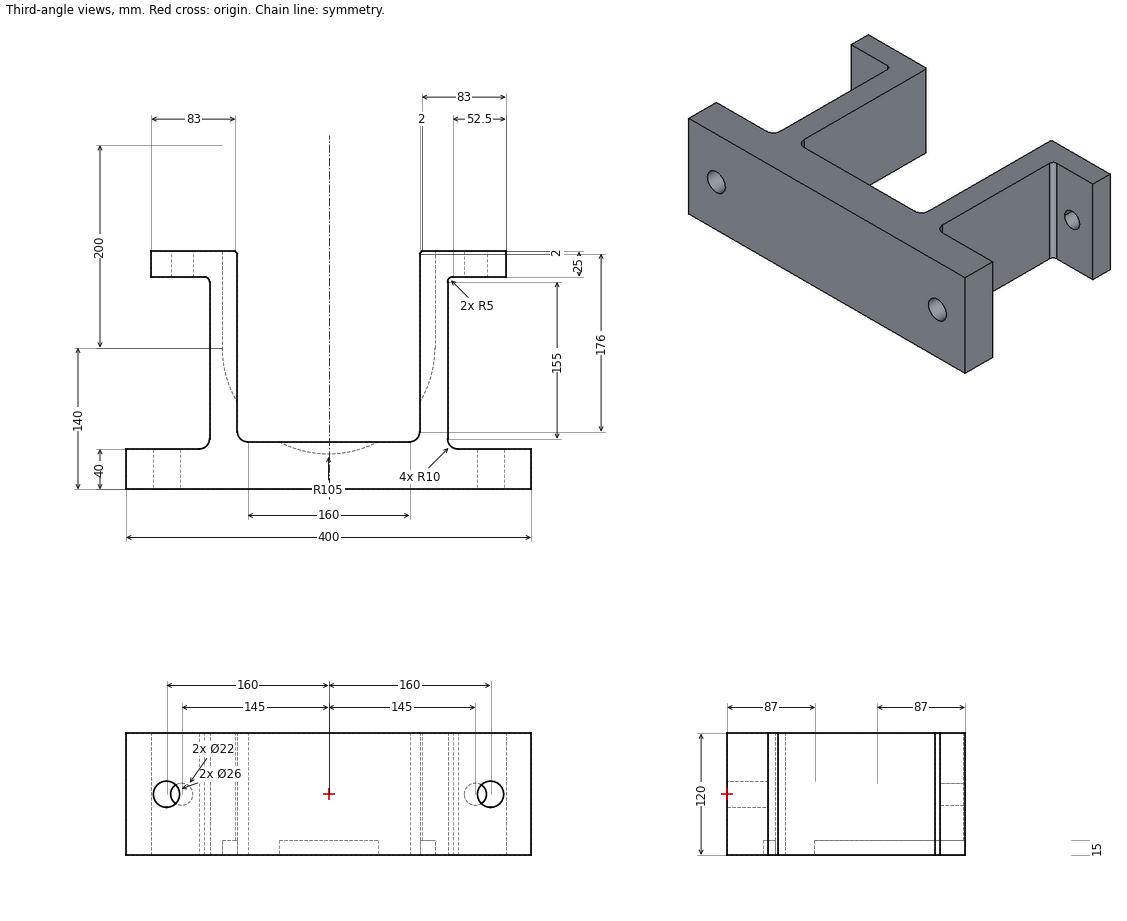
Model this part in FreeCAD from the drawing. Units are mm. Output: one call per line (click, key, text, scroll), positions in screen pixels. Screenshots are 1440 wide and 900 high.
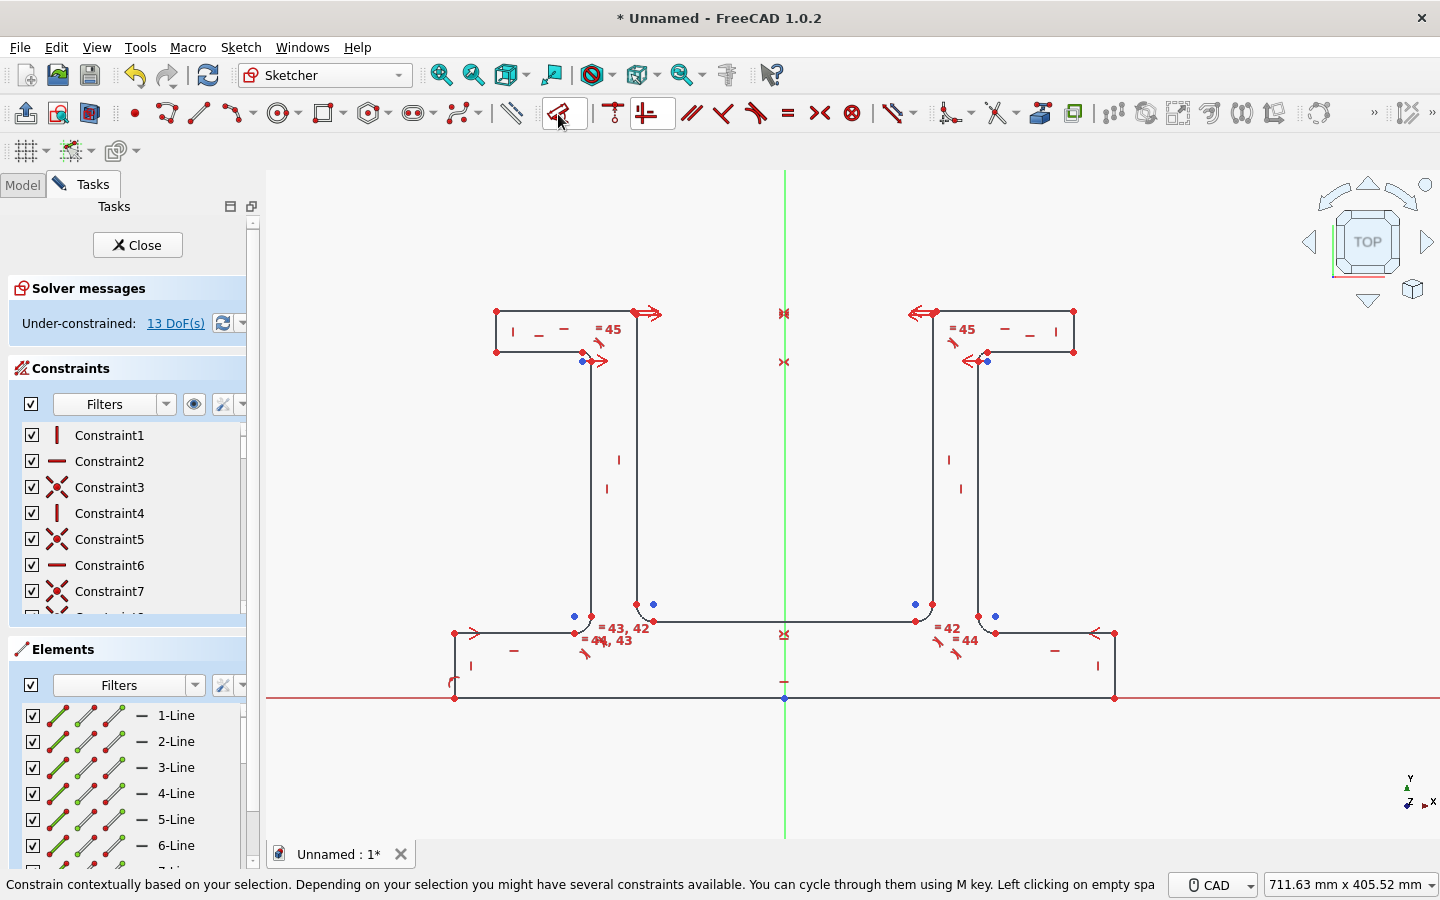
scroll(981, 355, up, 8)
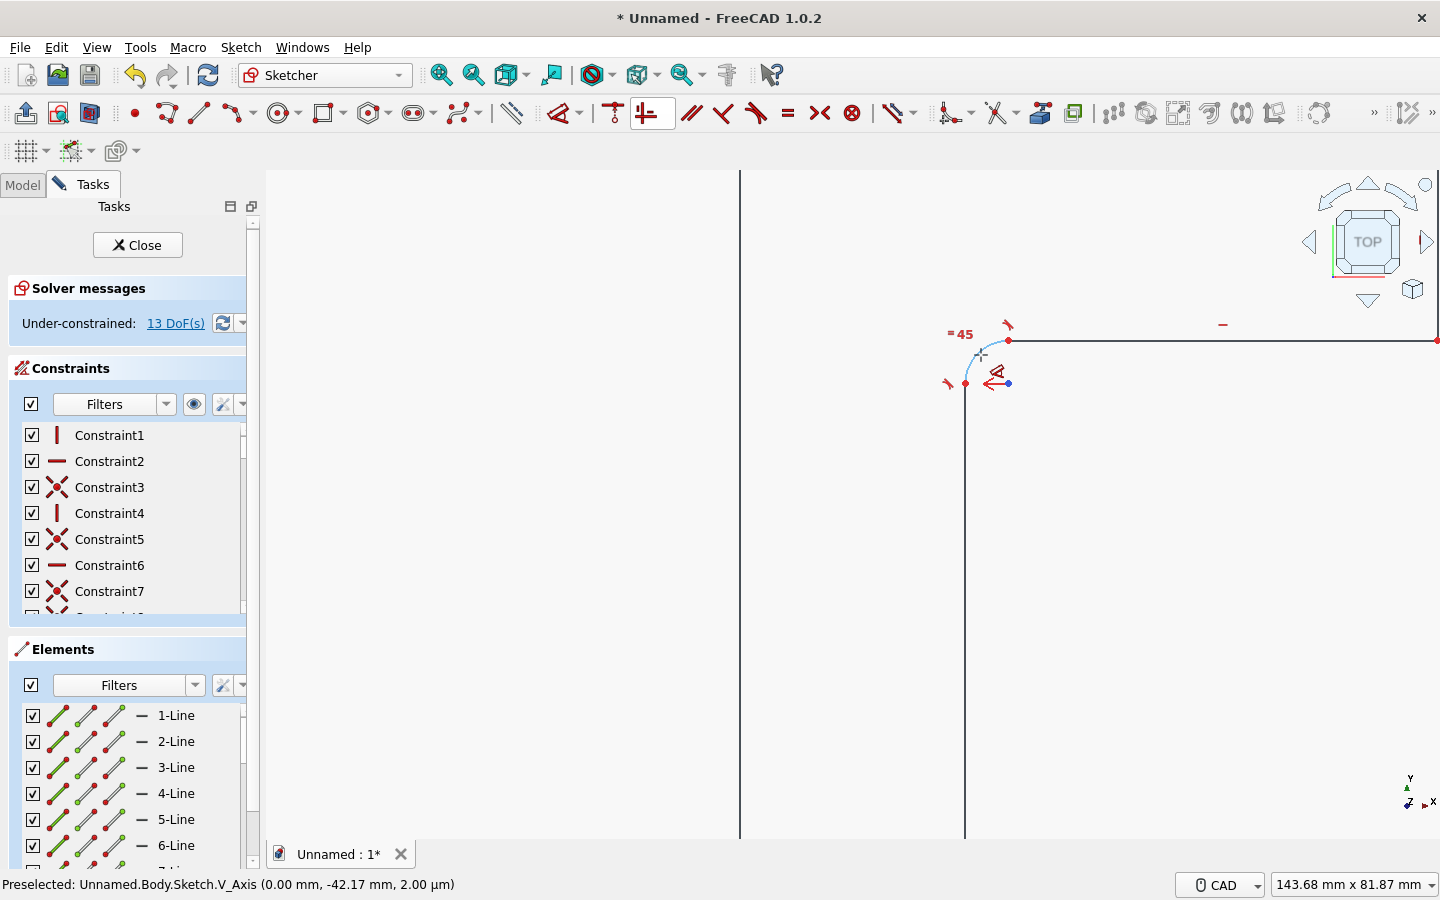
click(978, 354)
click(955, 332)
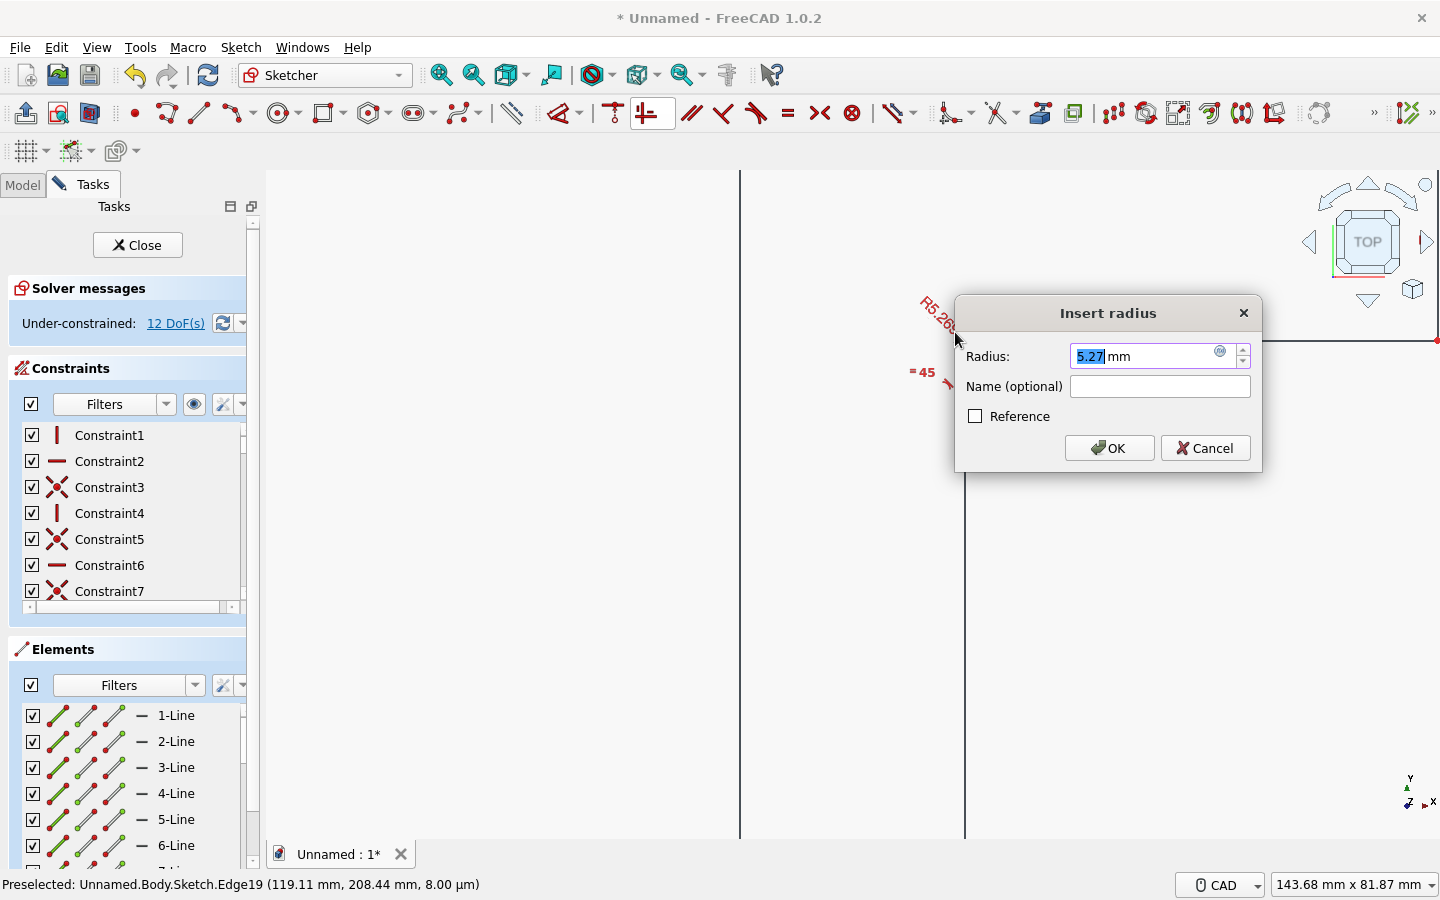
text(5)
key(Return)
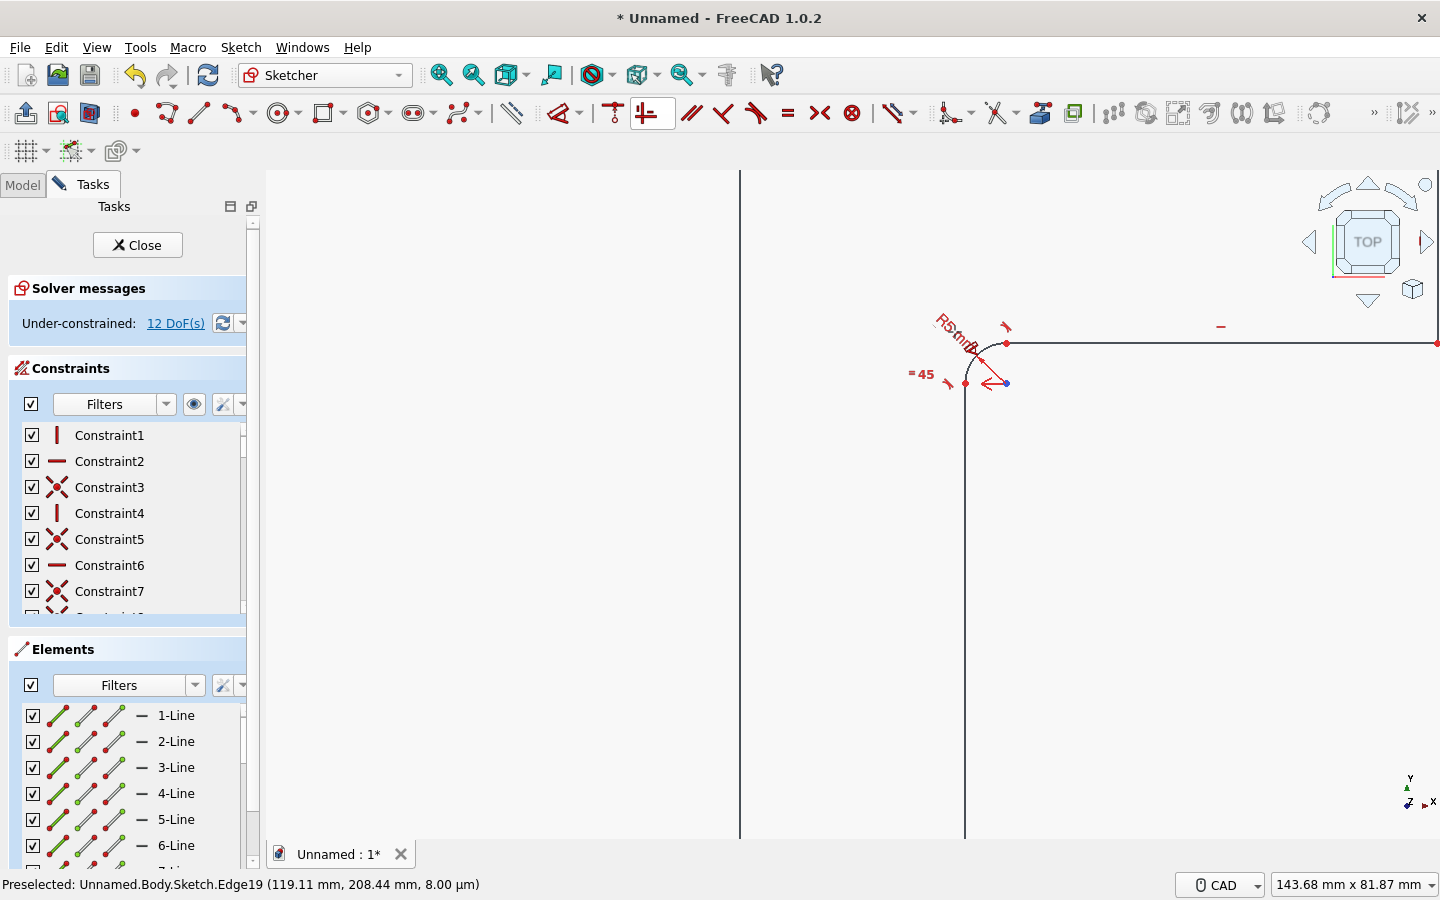
scroll(981, 355, down, 8)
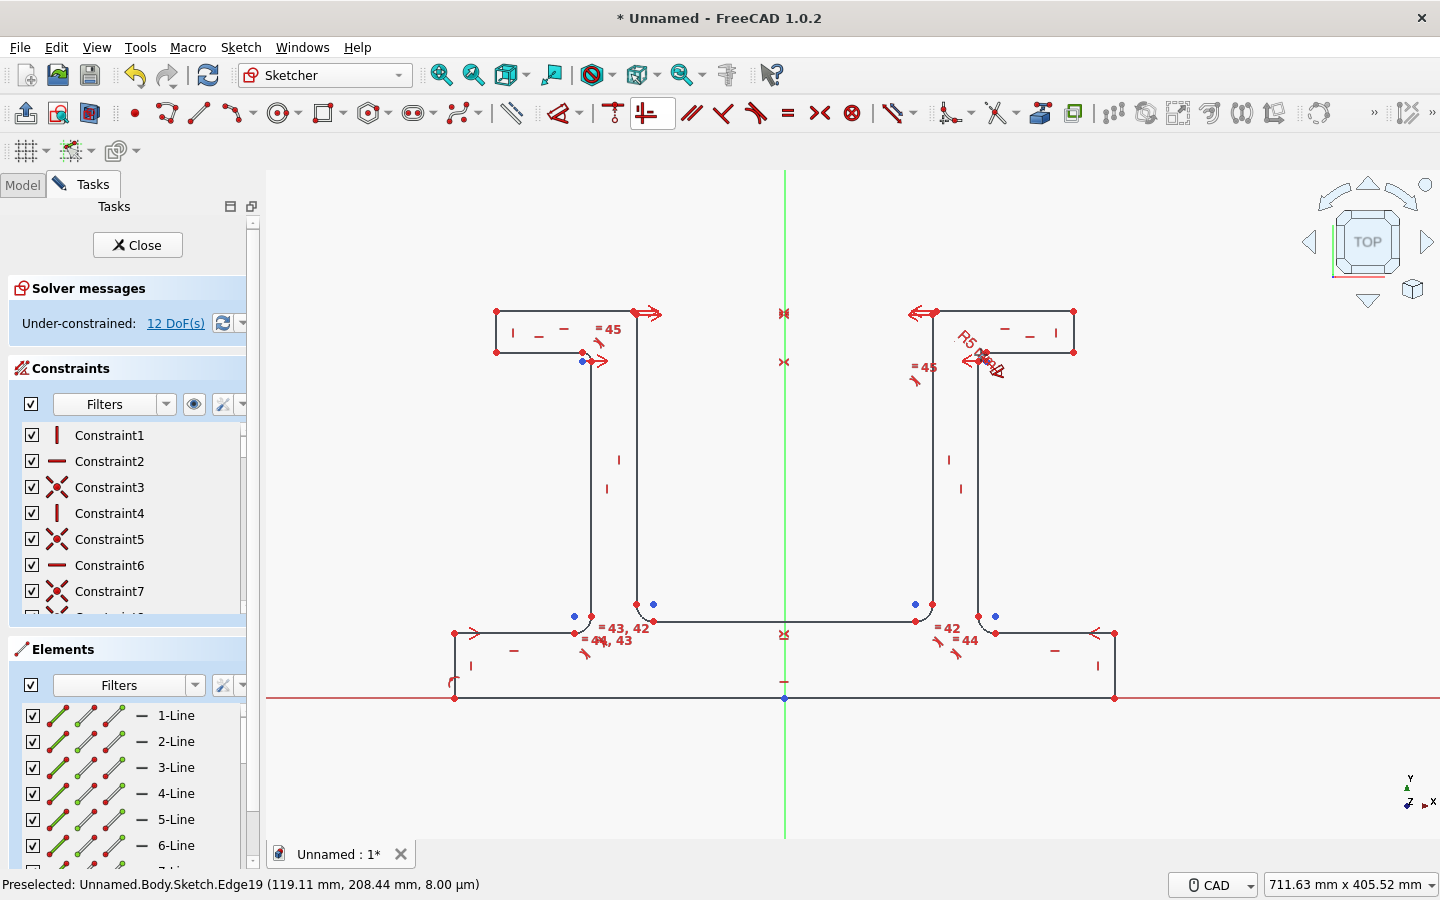
scroll(924, 620, up, 5)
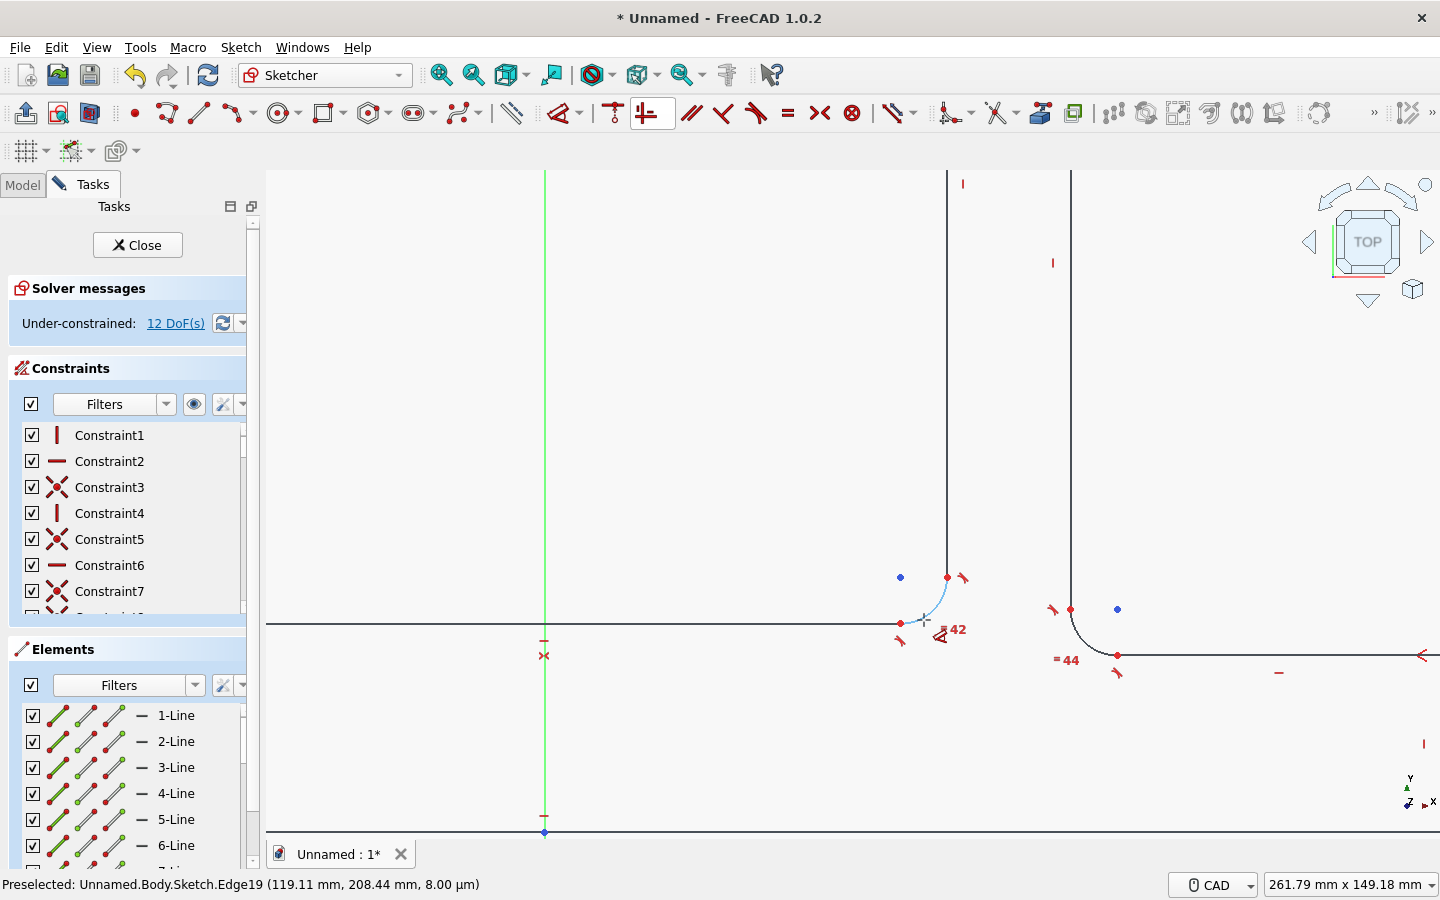
click(922, 619)
click(937, 647)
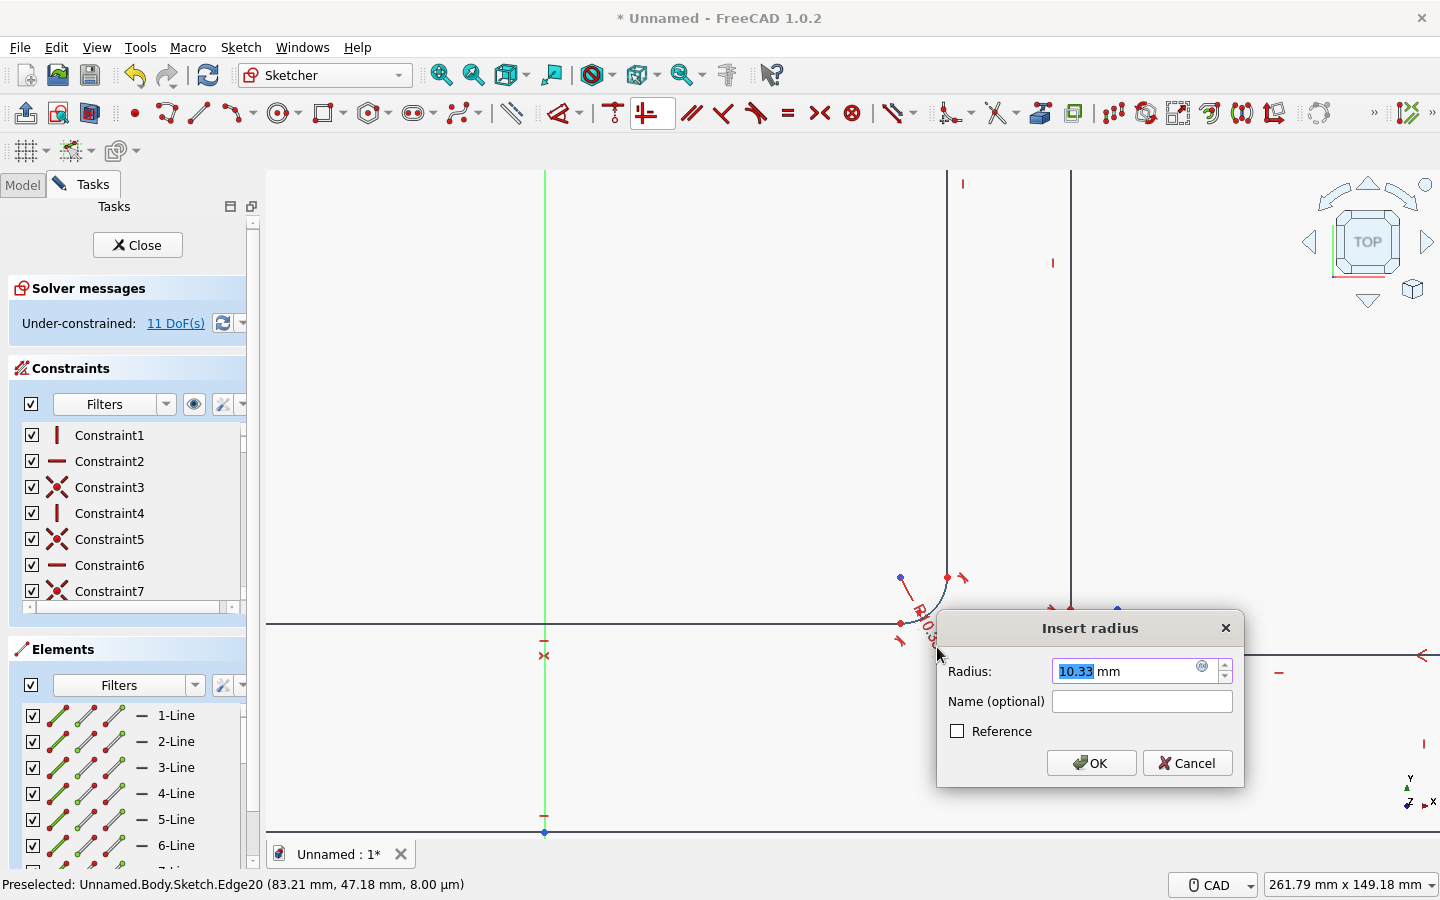
text(10)
key(Return)